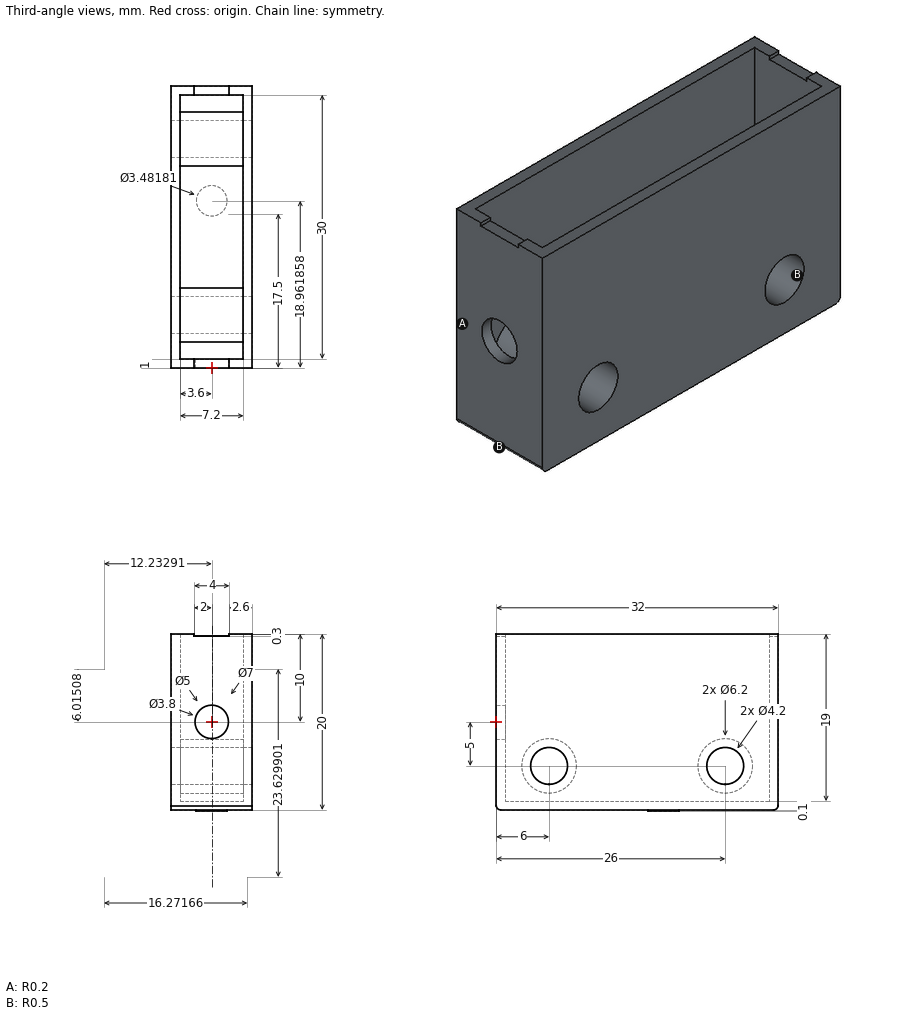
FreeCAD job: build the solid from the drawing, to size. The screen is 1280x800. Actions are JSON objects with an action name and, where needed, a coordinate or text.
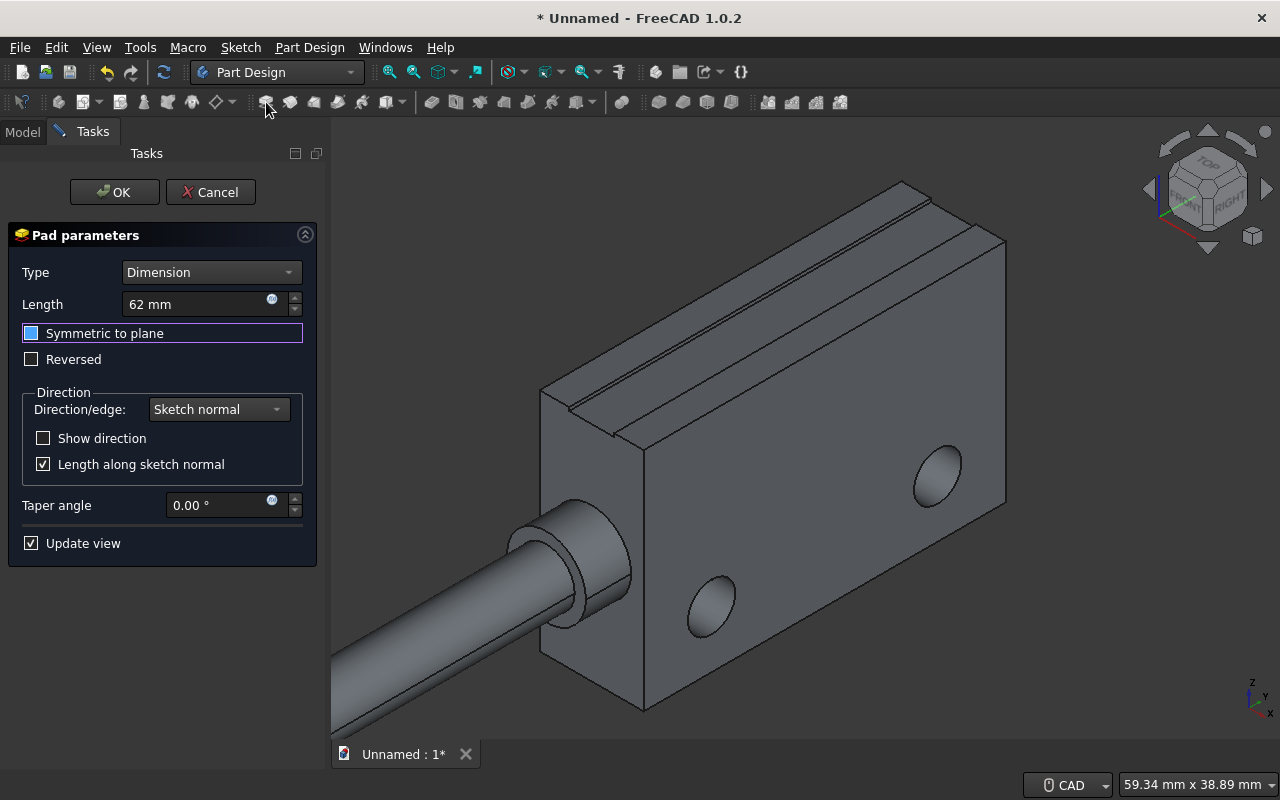
{"action": "left_click", "coordinate": [115, 192]}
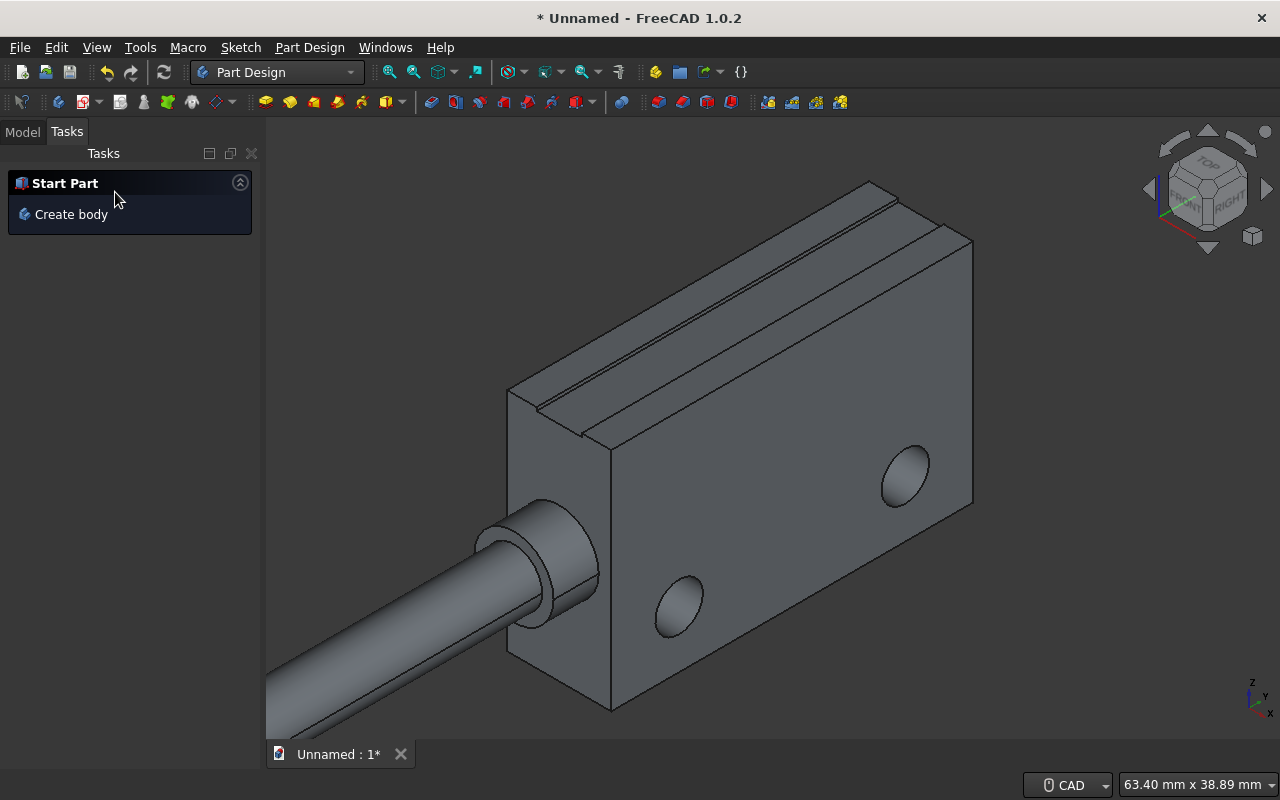
{"action": "left_click", "coordinate": [390, 72]}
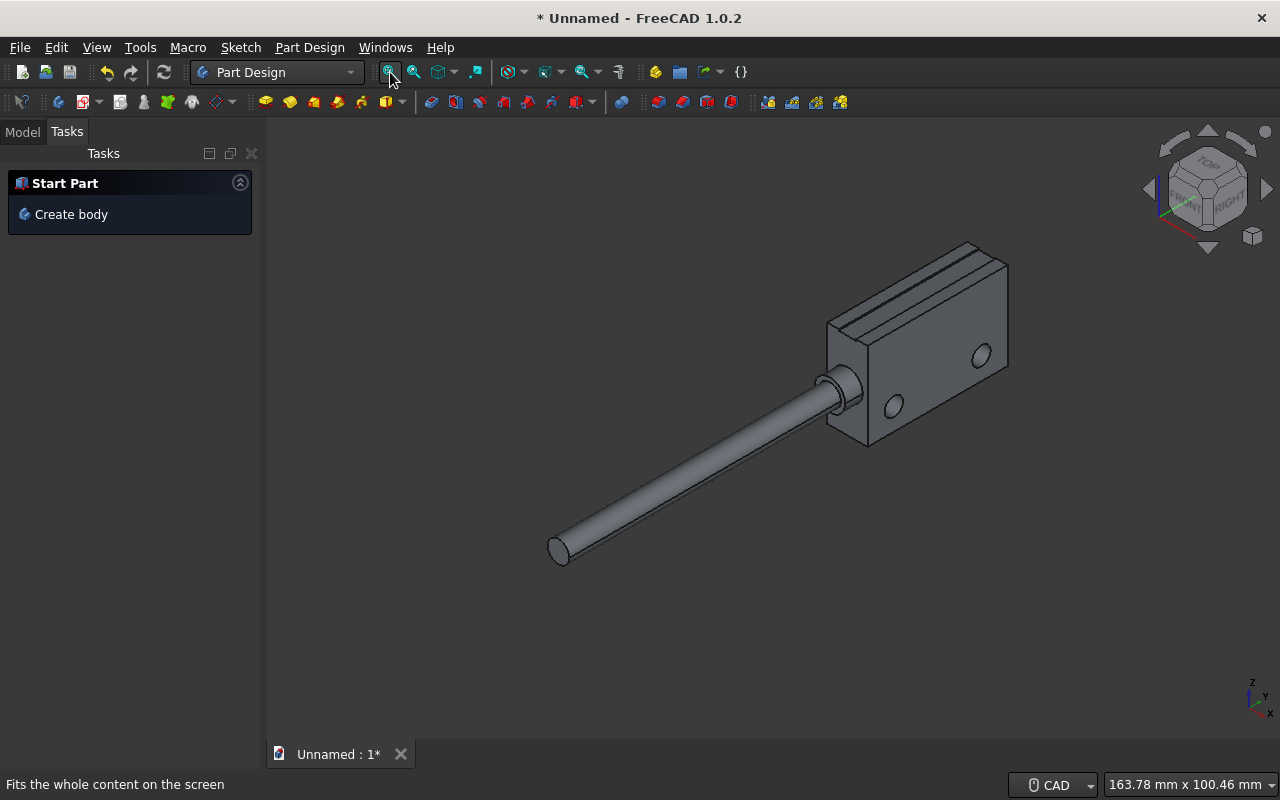
{"action": "left_click", "coordinate": [818, 376]}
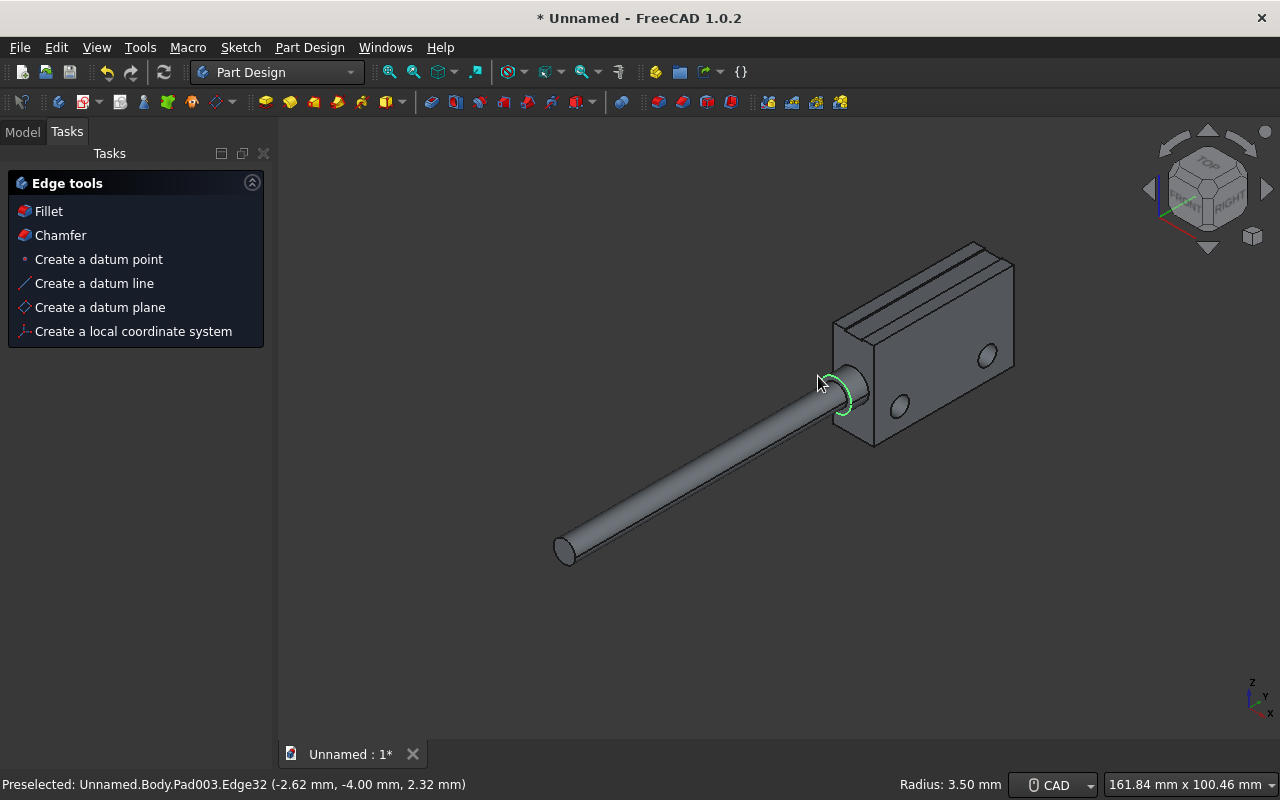
{"action": "left_click", "coordinate": [660, 102]}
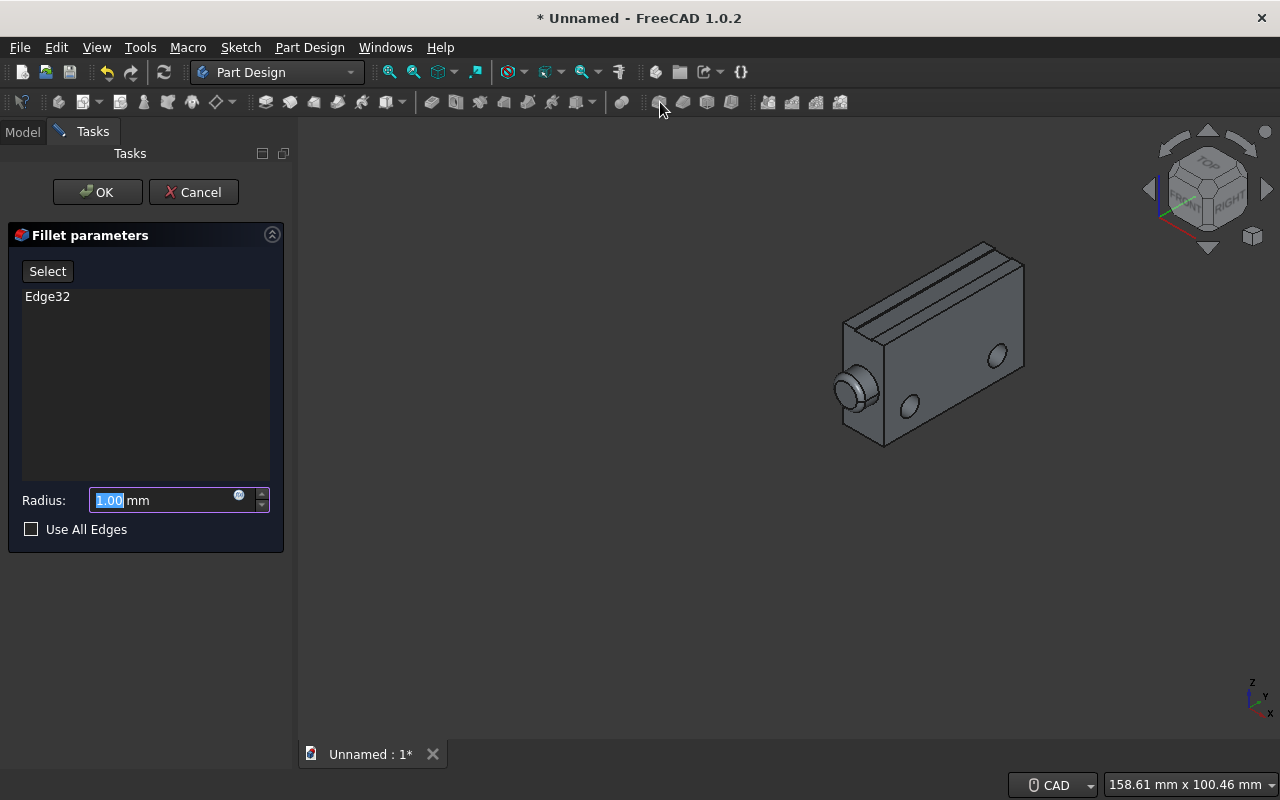
{"action": "type", "text": "0.2"}
{"action": "key", "text": "Tab"}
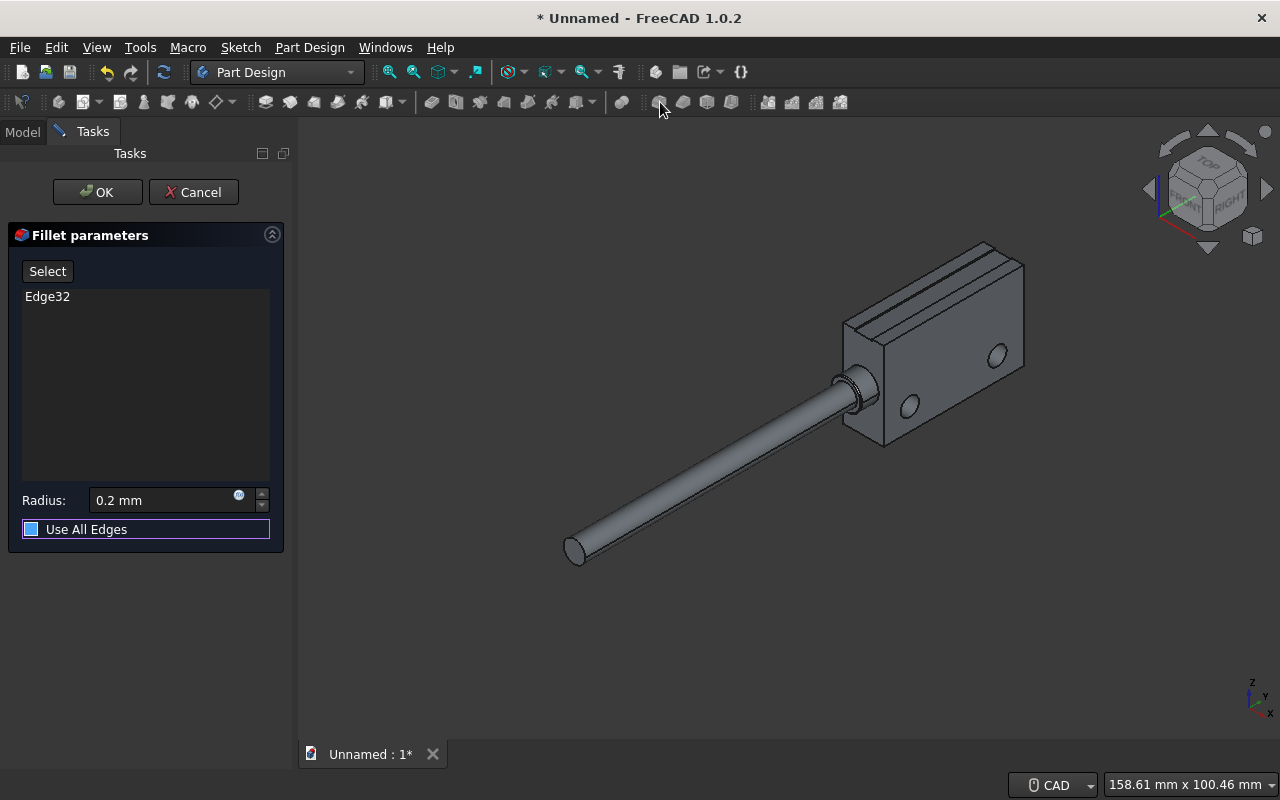
{"action": "left_click", "coordinate": [98, 192]}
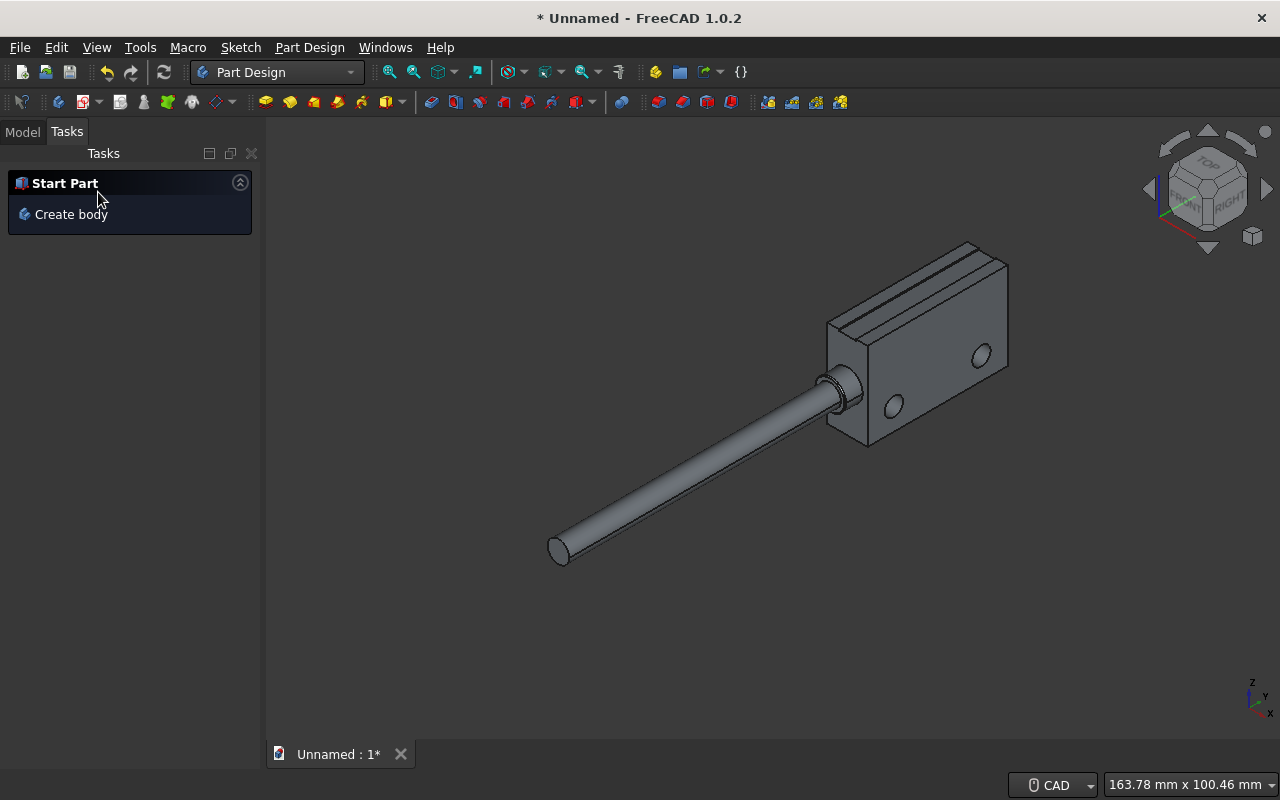
{"action": "key", "text": "2"}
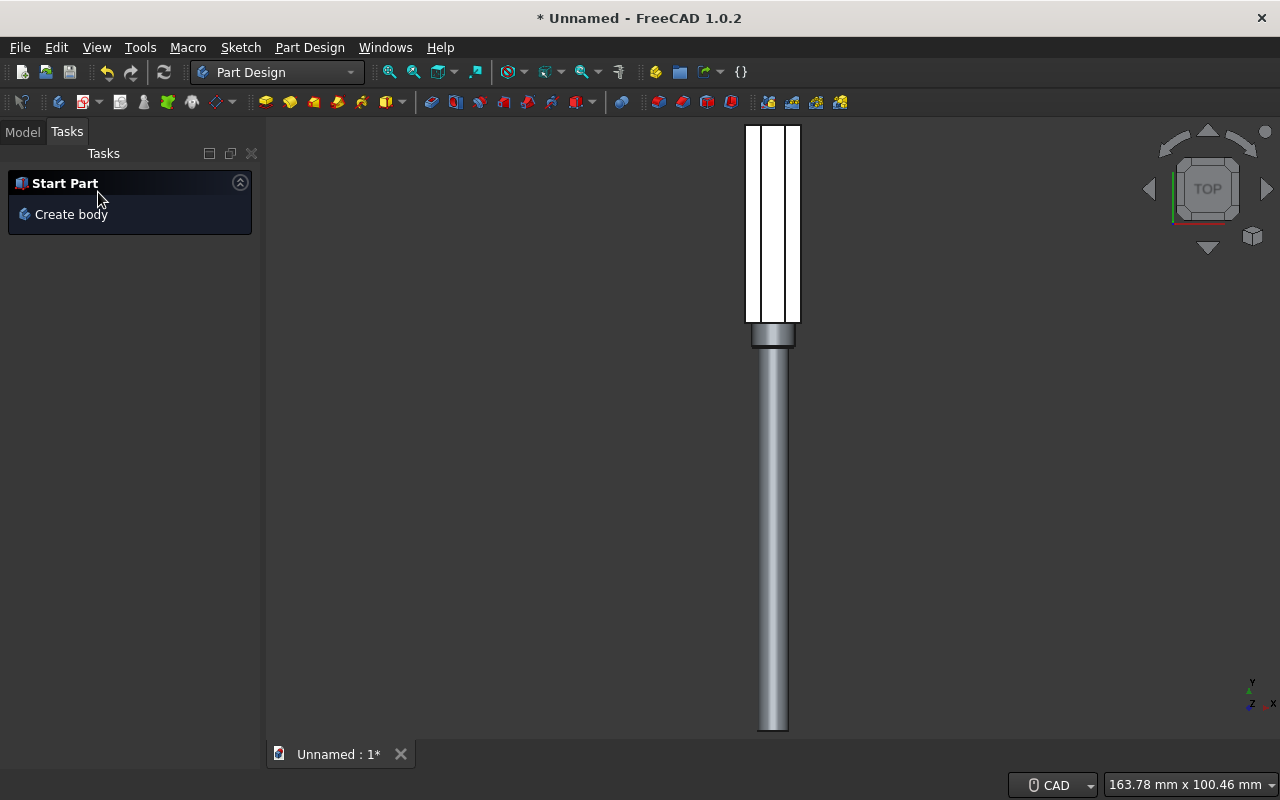
{"action": "key", "text": "0"}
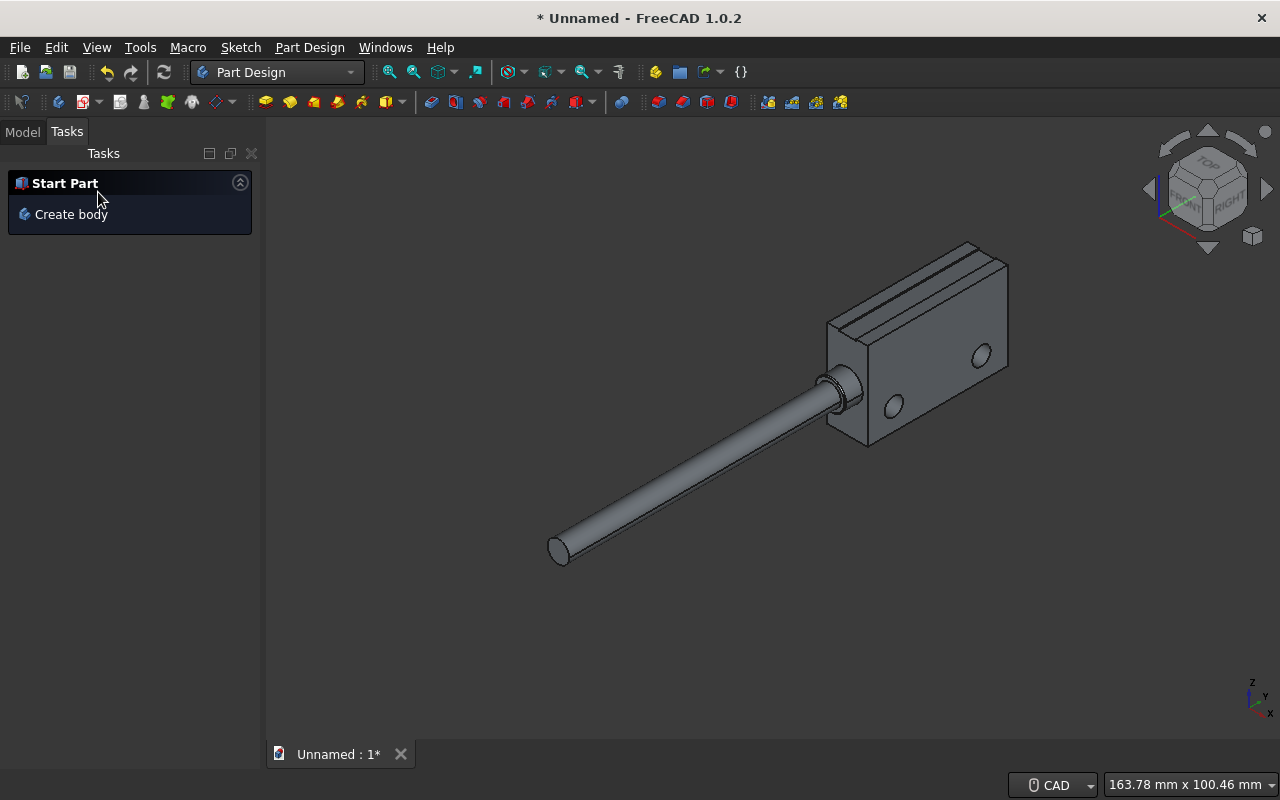
{"action": "key", "text": "1"}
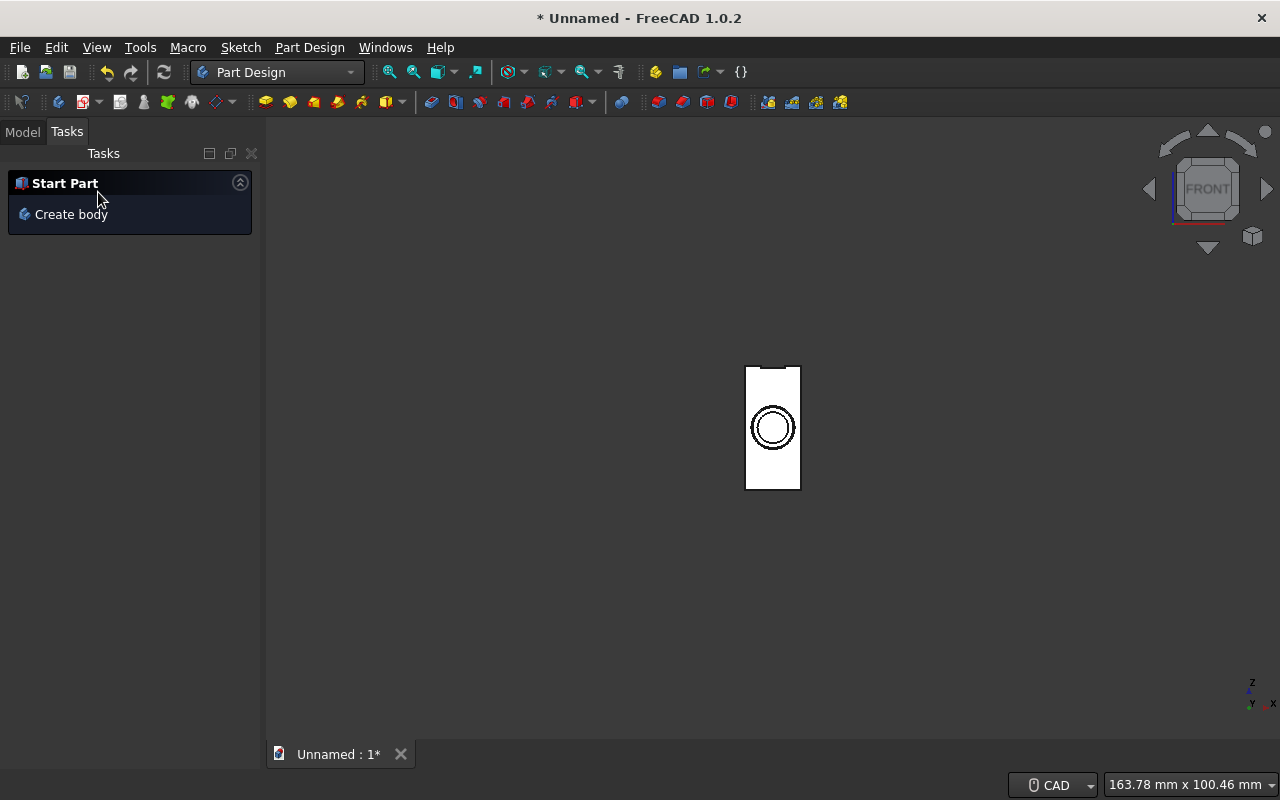
{"action": "left_click", "coordinate": [390, 72]}